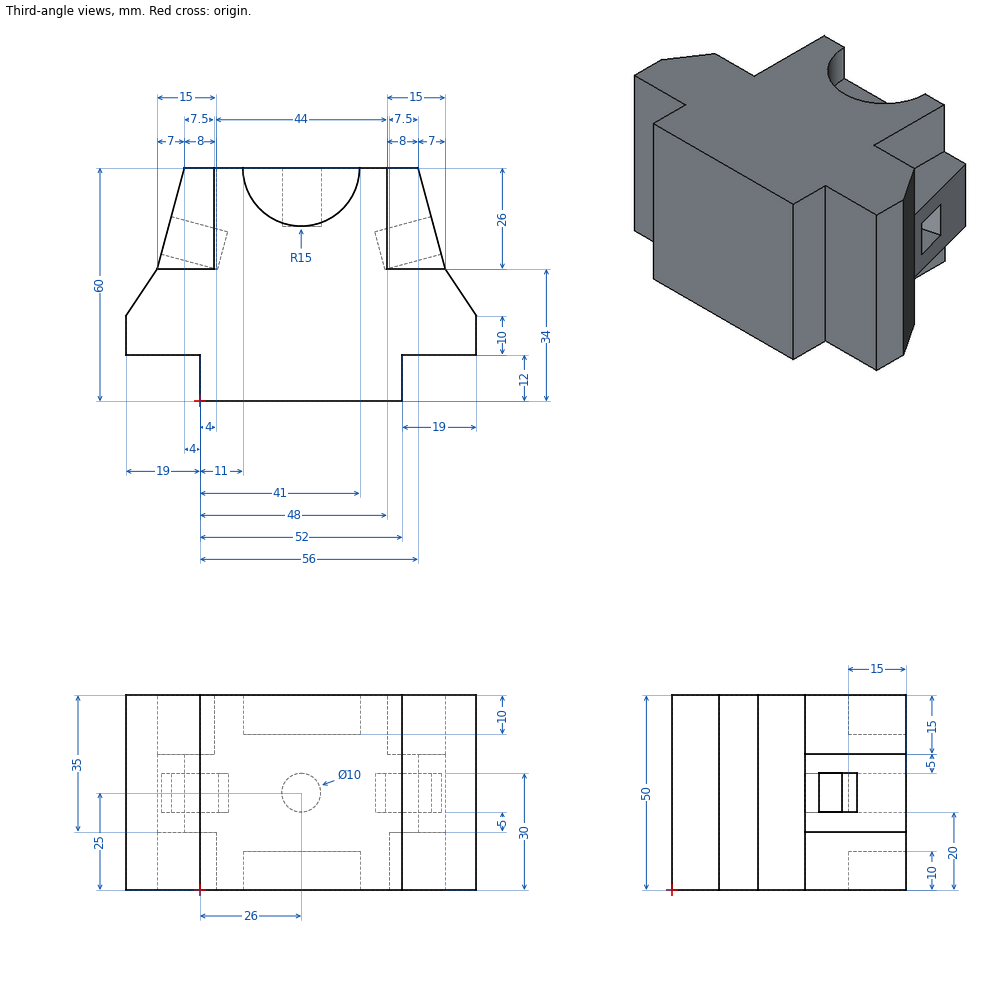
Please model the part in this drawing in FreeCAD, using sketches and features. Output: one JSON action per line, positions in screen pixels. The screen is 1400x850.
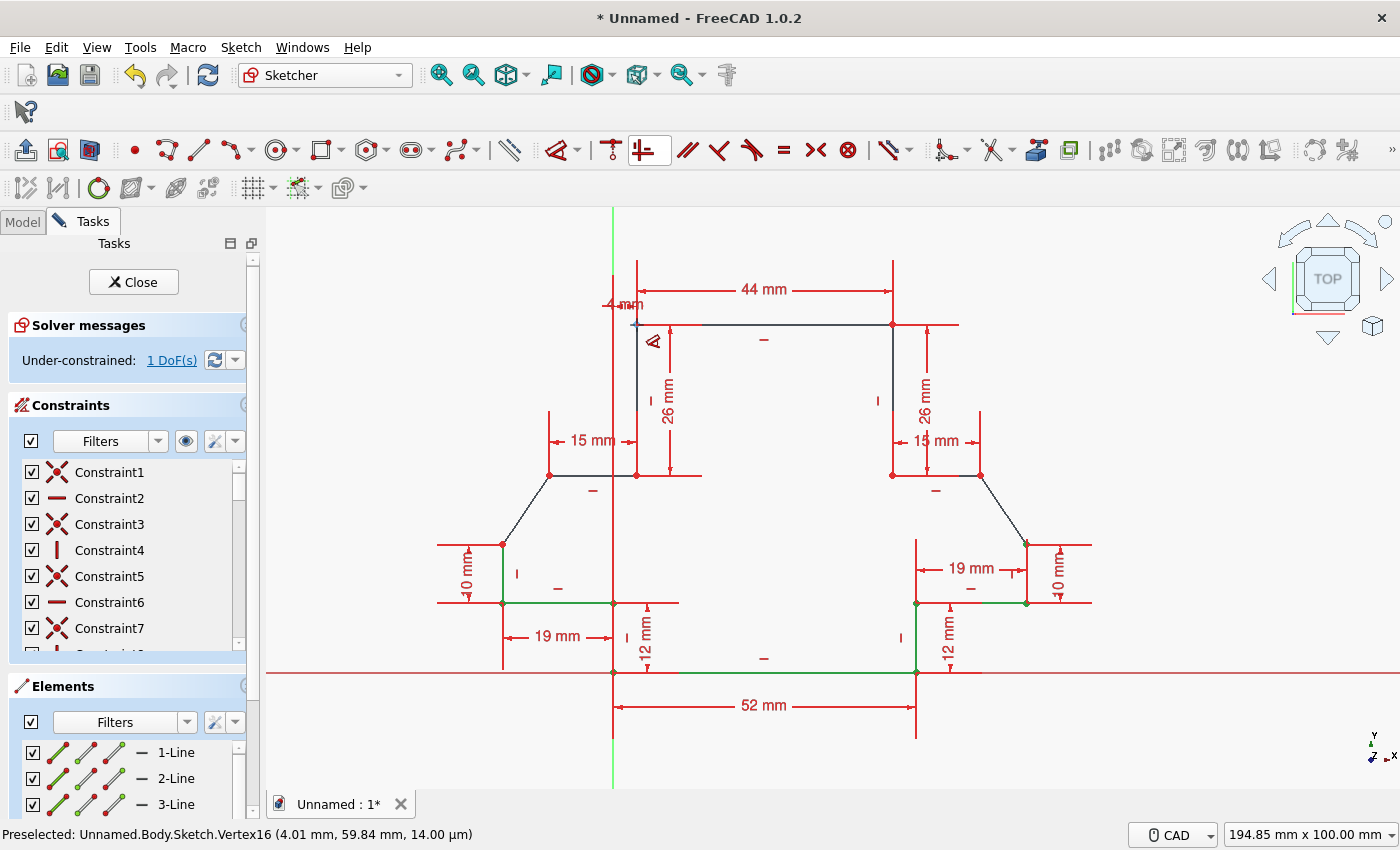
{"action": "left_click", "coordinate": [980, 476]}
{"action": "left_click", "coordinate": [579, 574]}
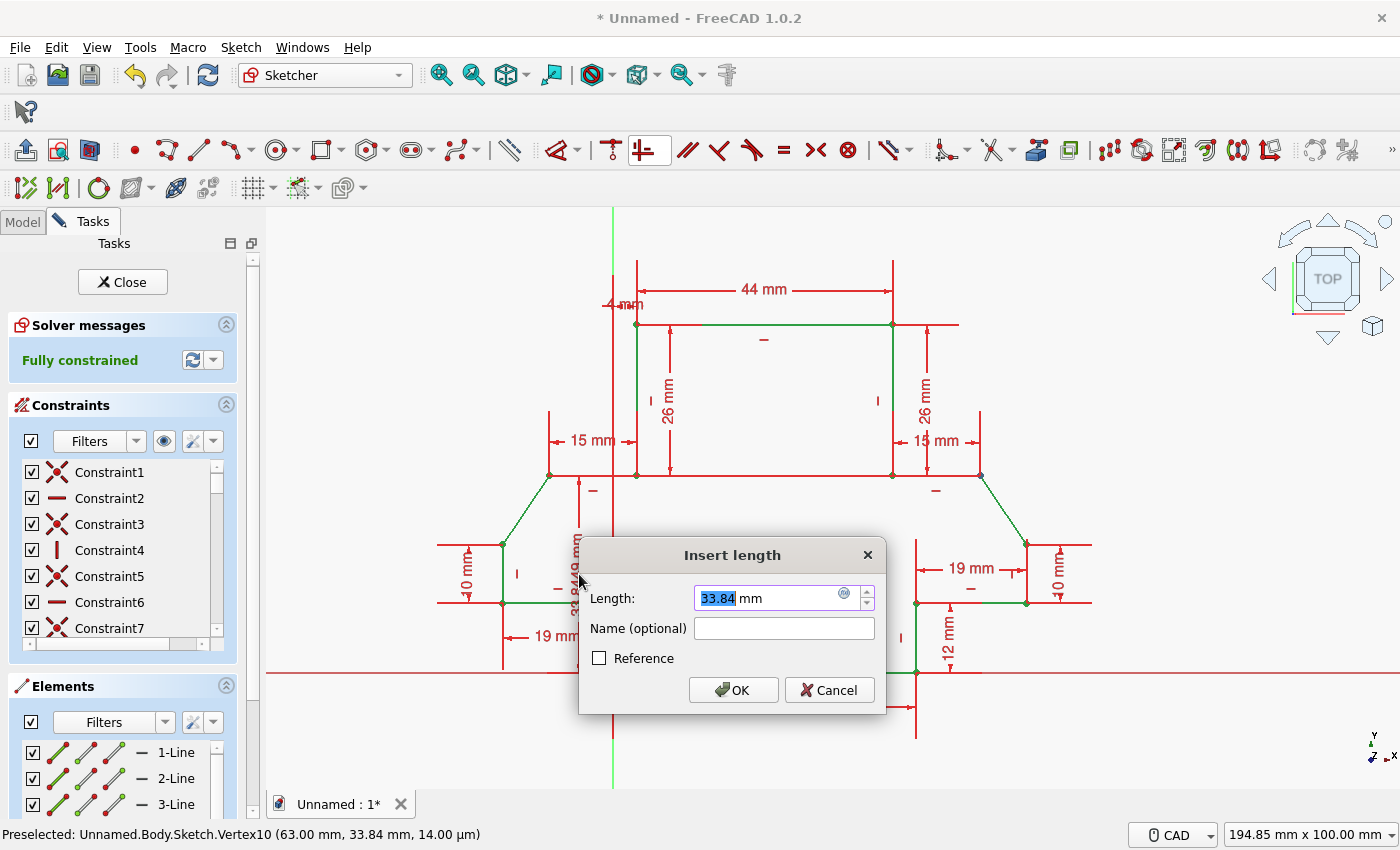
{"action": "type", "text": "34"}
{"action": "key", "text": "Return"}
{"action": "key", "text": "Escape"}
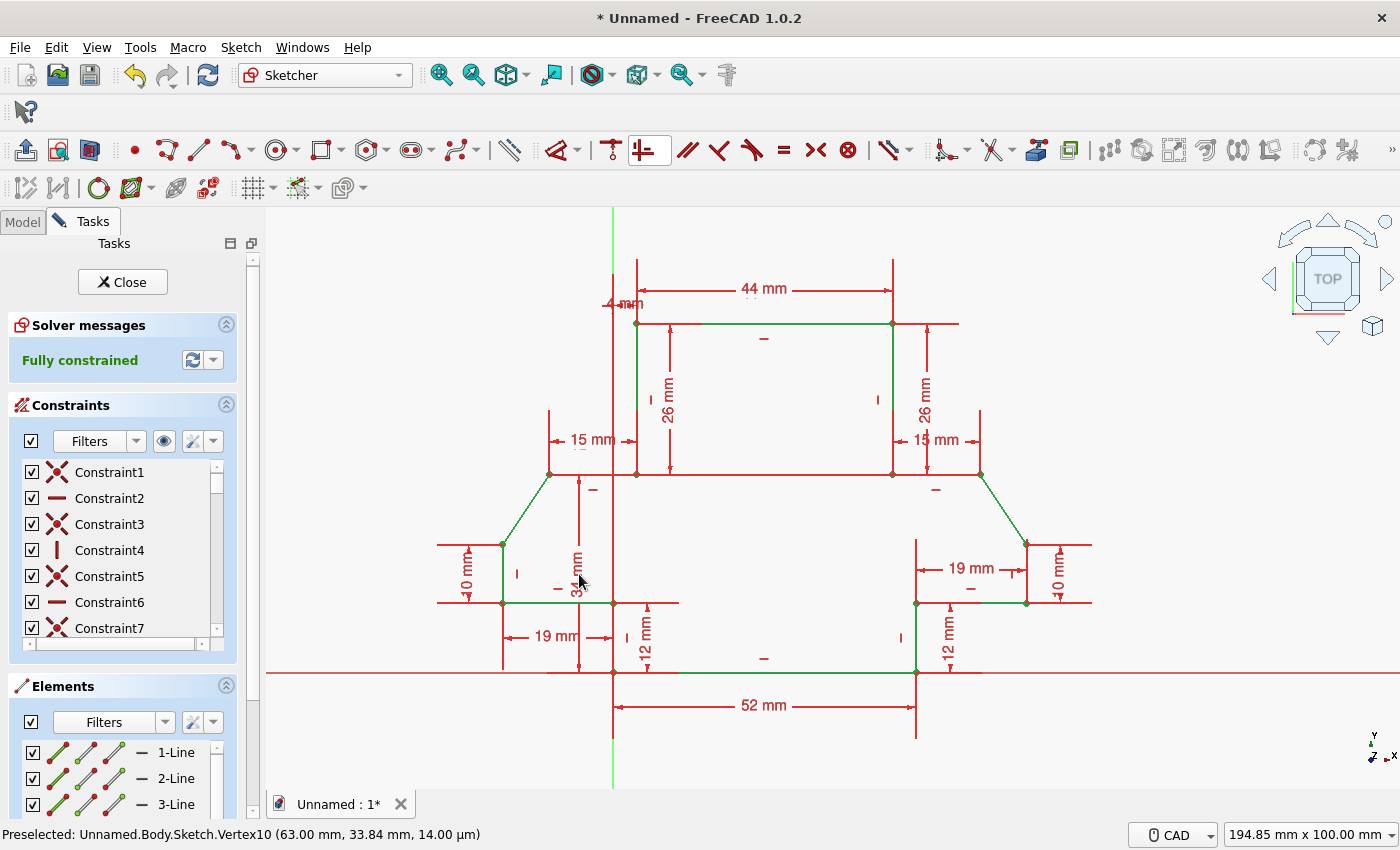
{"action": "left_click", "coordinate": [123, 282]}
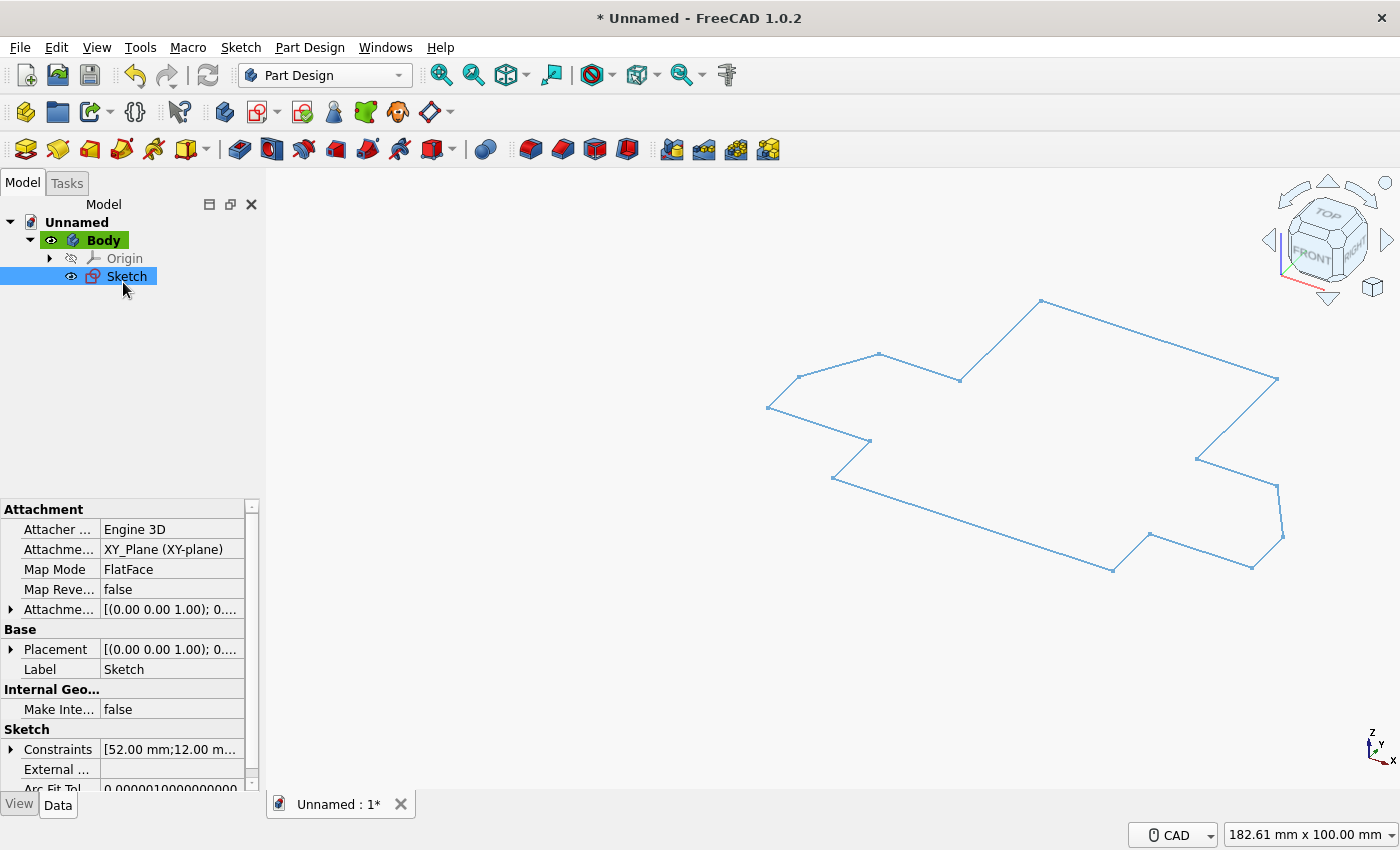
{"action": "left_click", "coordinate": [26, 150]}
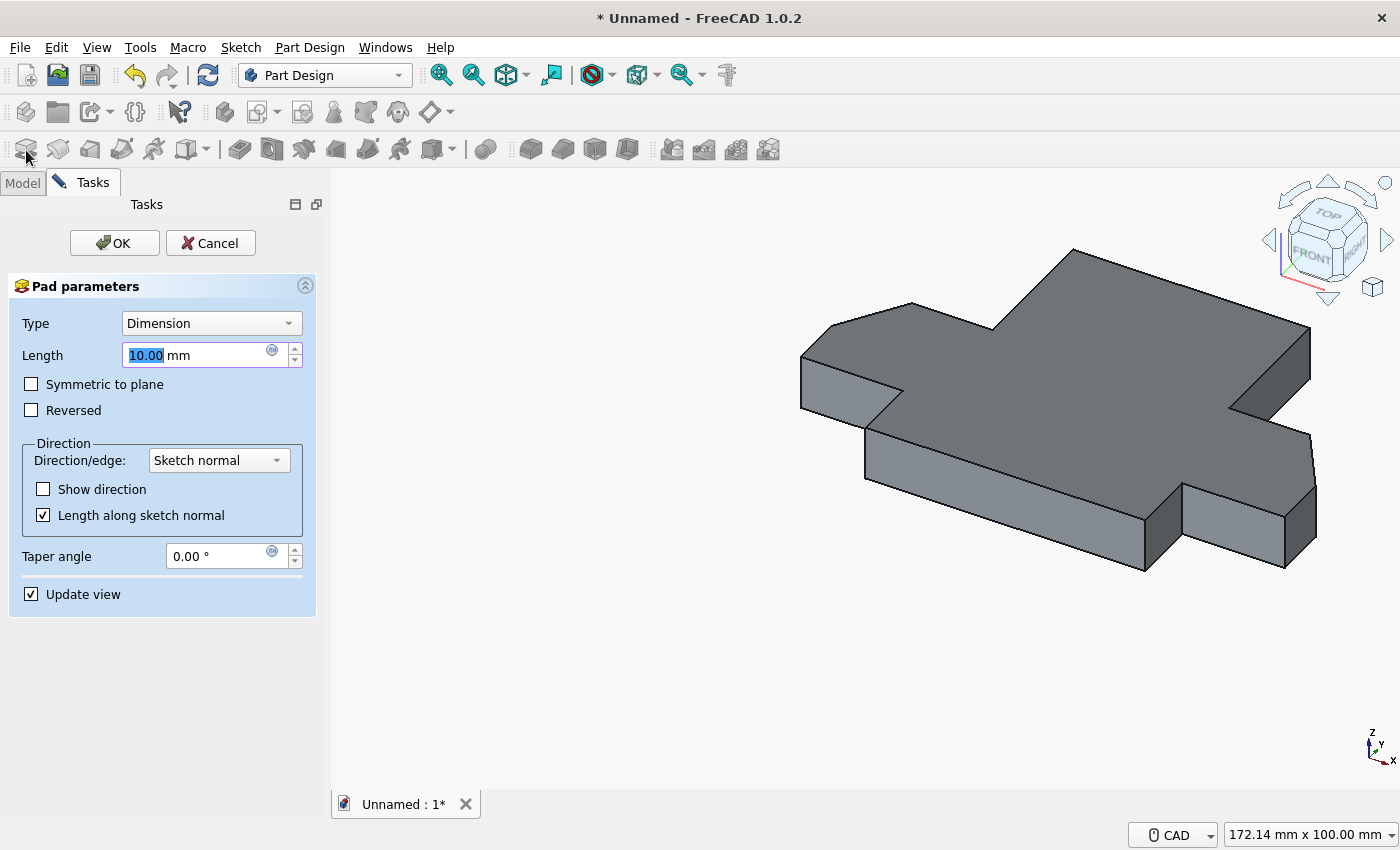
{"action": "type", "text": "50"}
{"action": "key", "text": "Tab"}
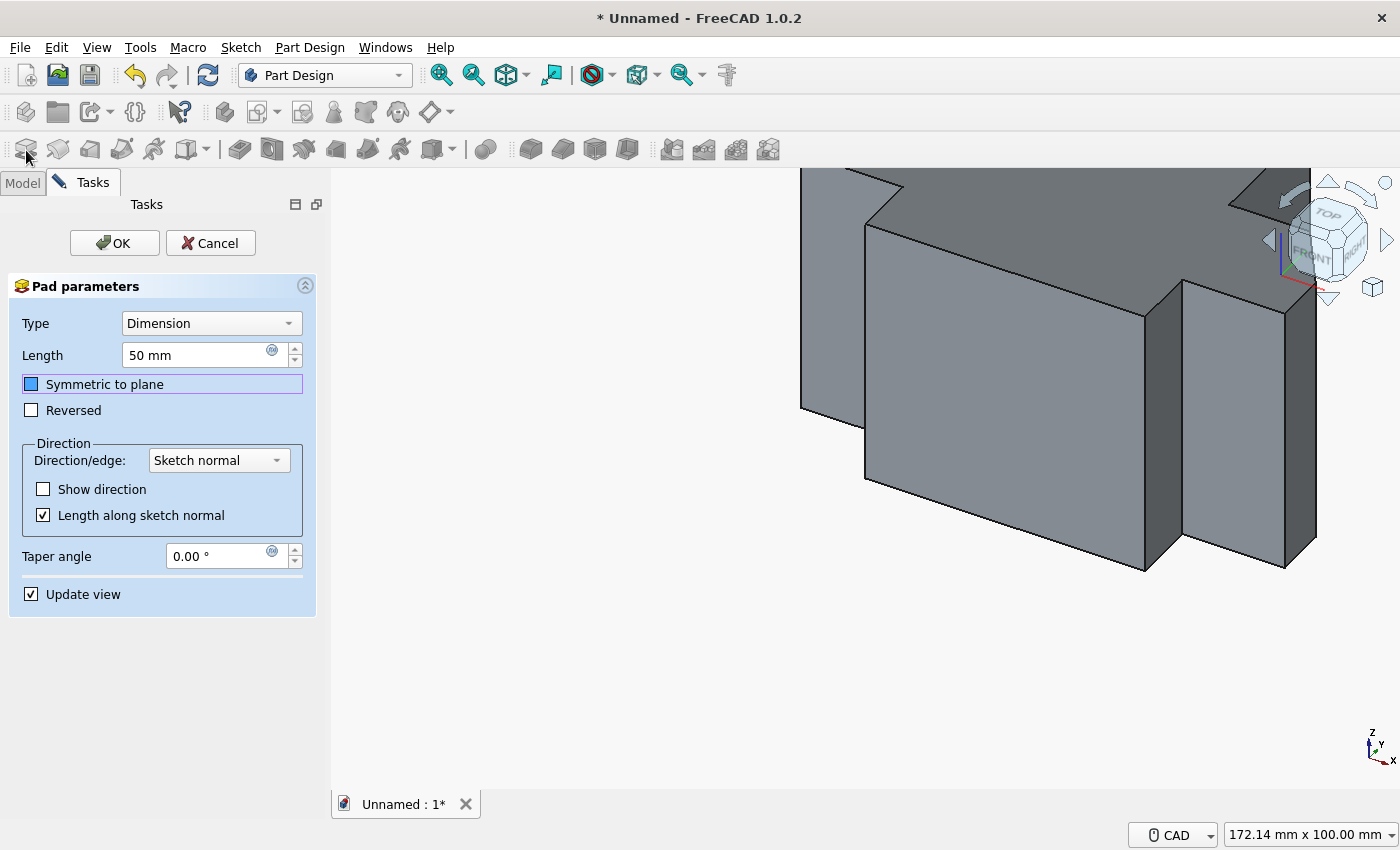
{"action": "left_click", "coordinate": [115, 243]}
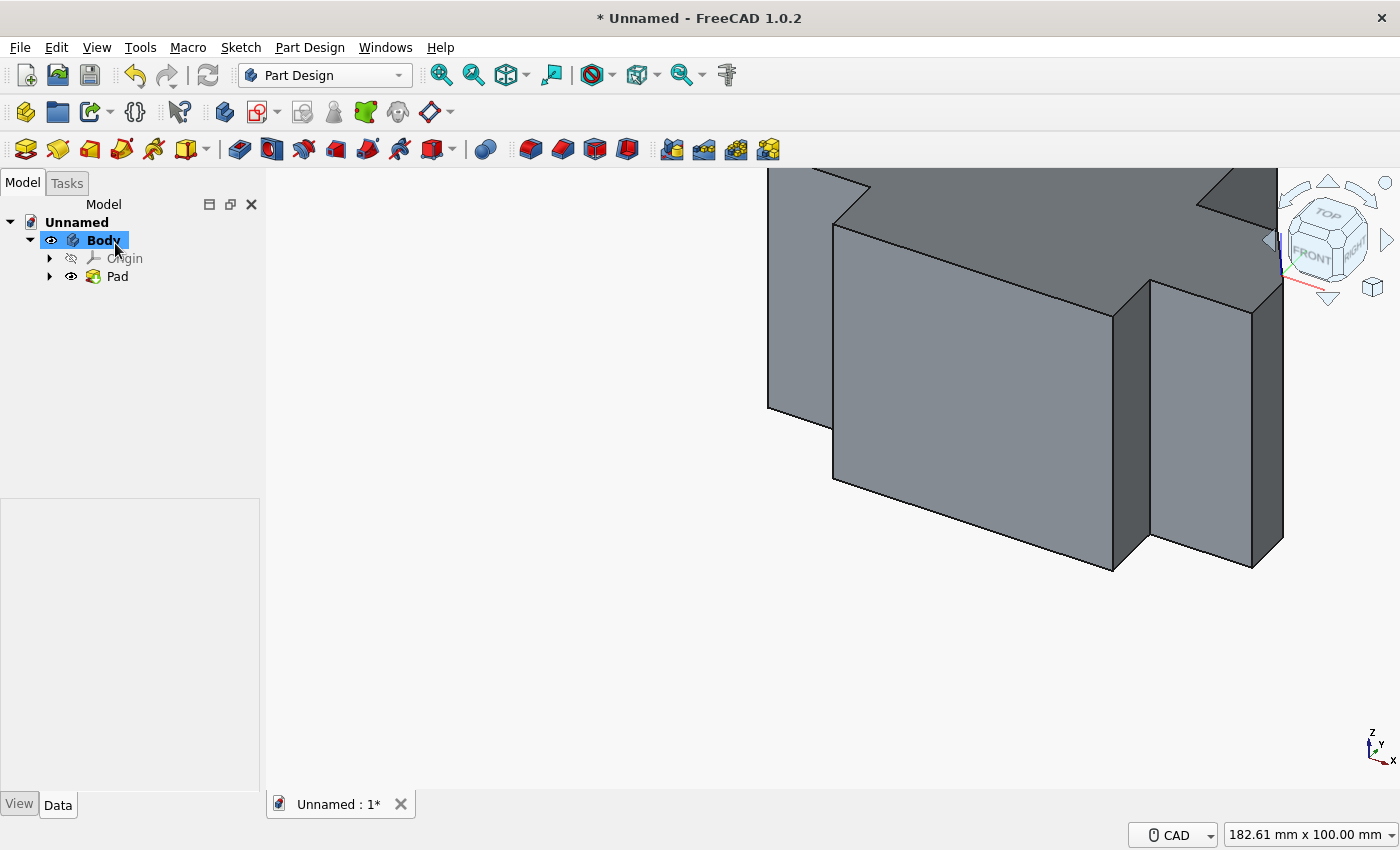
{"action": "left_click", "coordinate": [442, 76]}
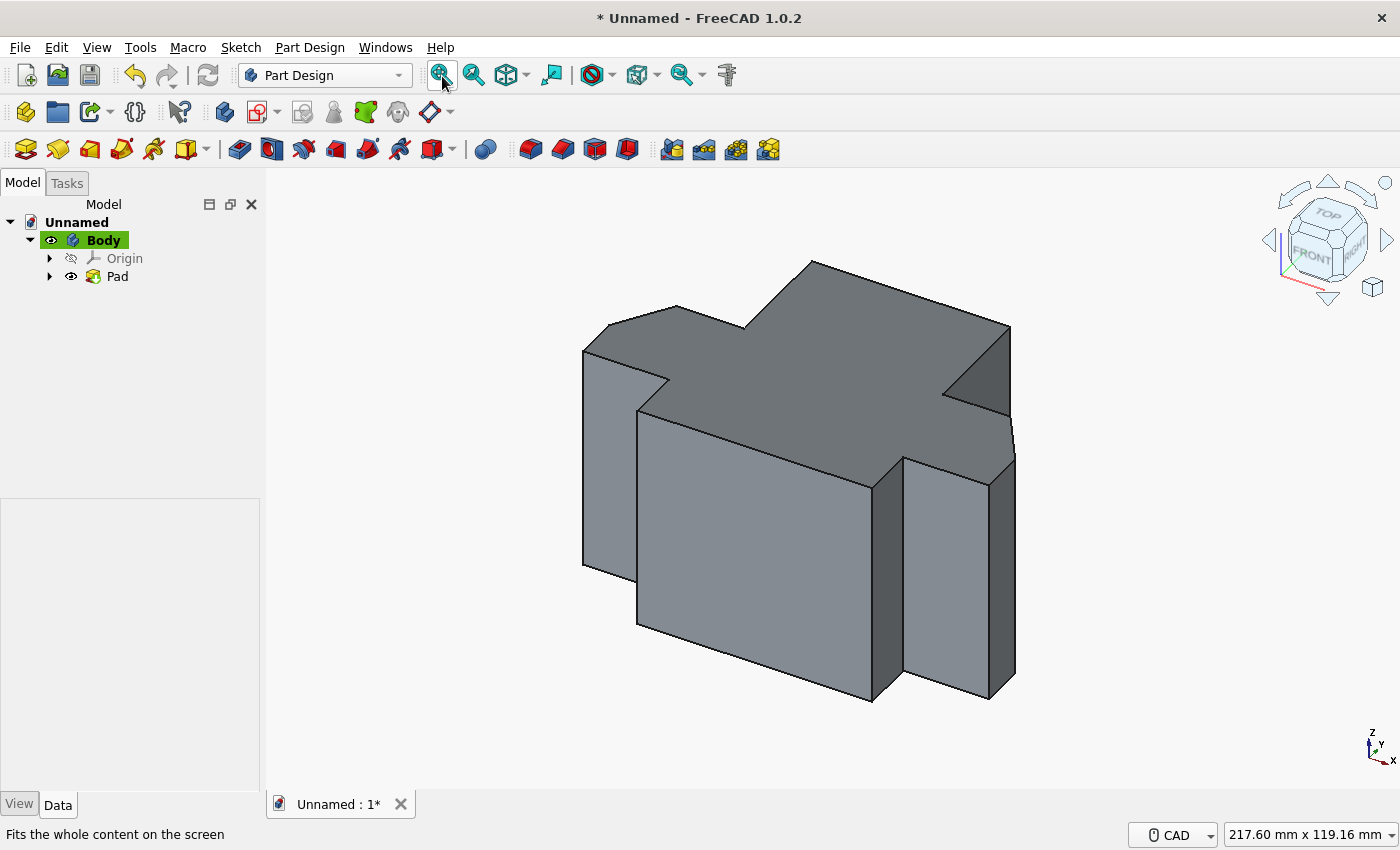
{"action": "left_click", "coordinate": [833, 371]}